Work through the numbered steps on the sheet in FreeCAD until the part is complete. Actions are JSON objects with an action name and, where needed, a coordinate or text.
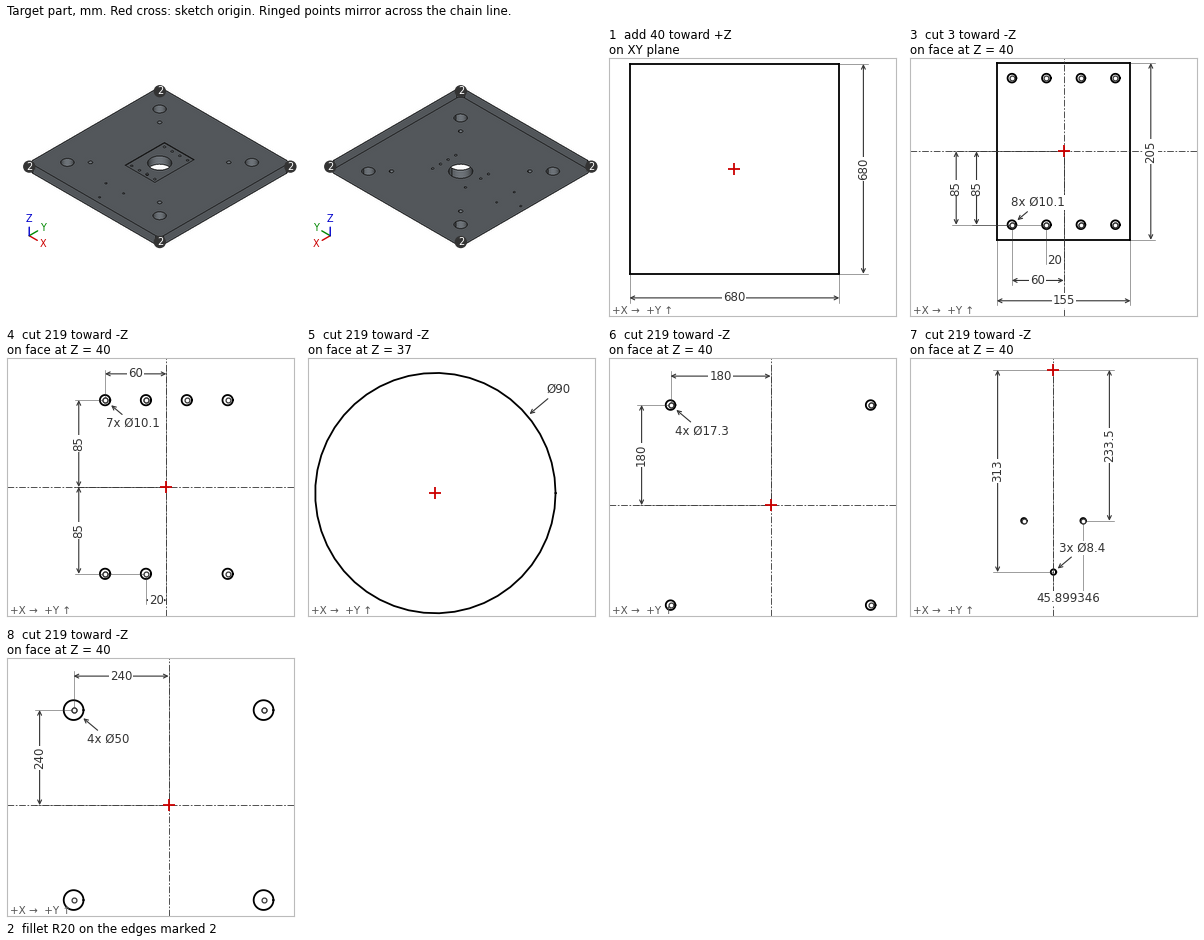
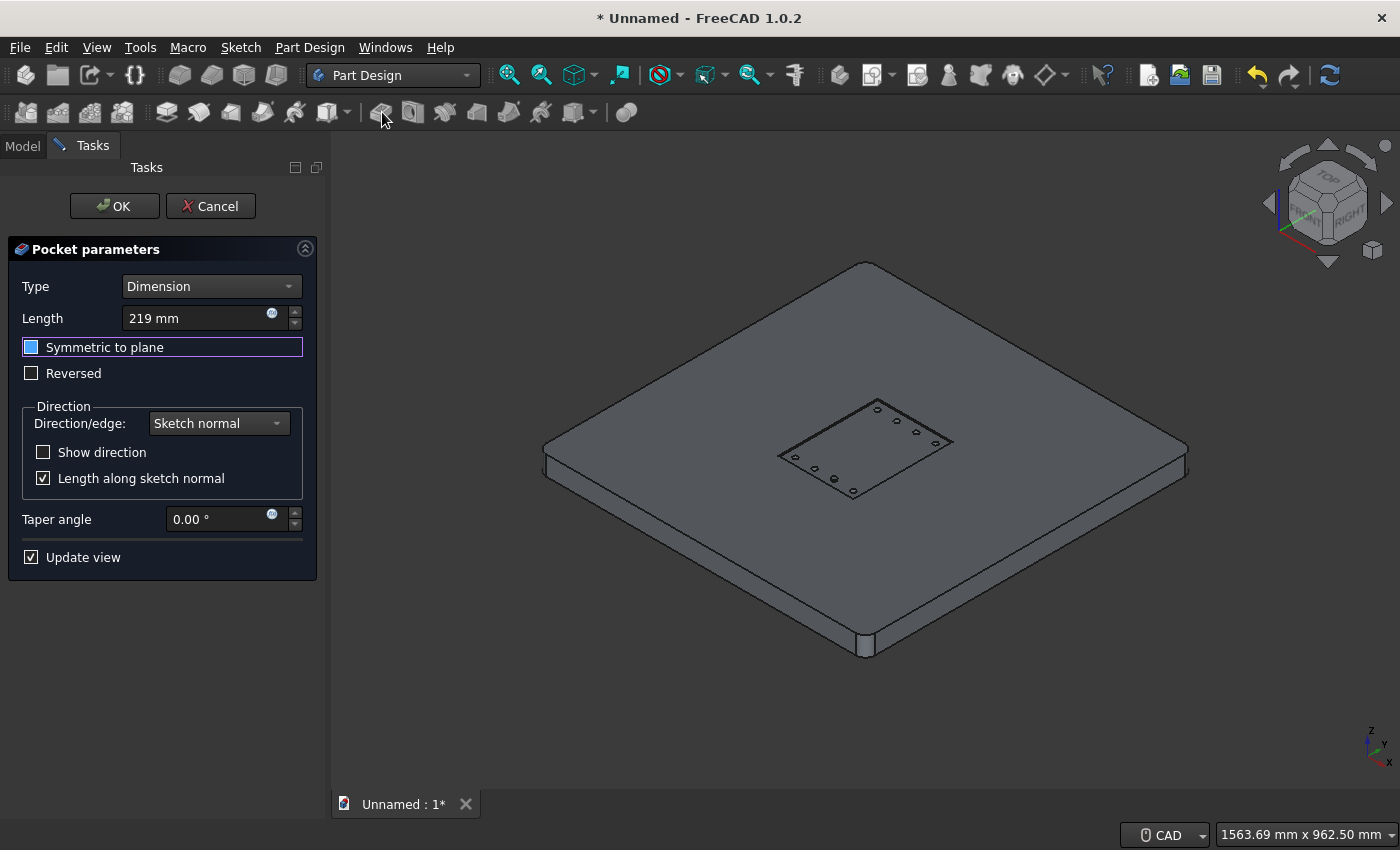
{"action": "left_click", "coordinate": [115, 206]}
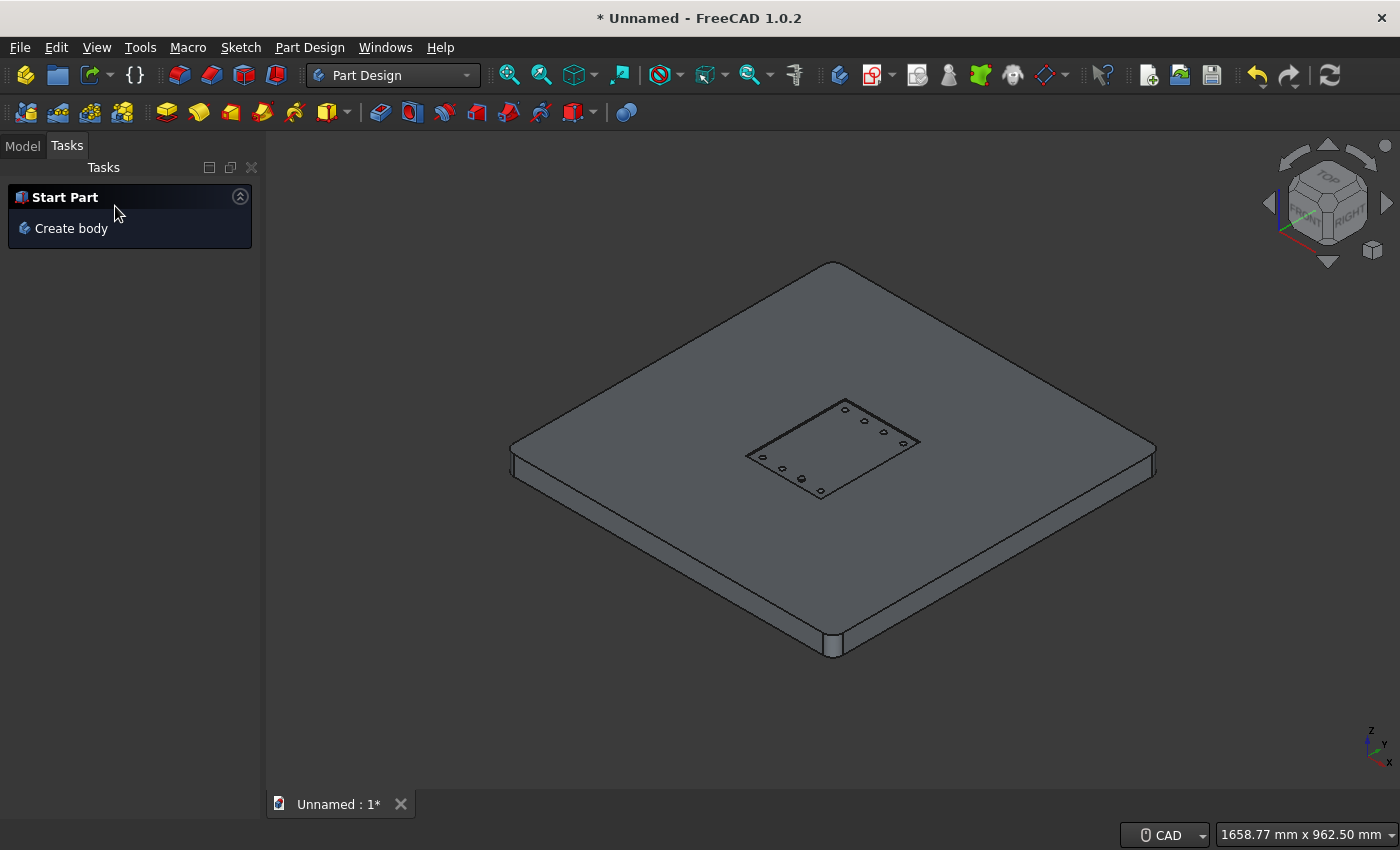
{"action": "left_click", "coordinate": [833, 450]}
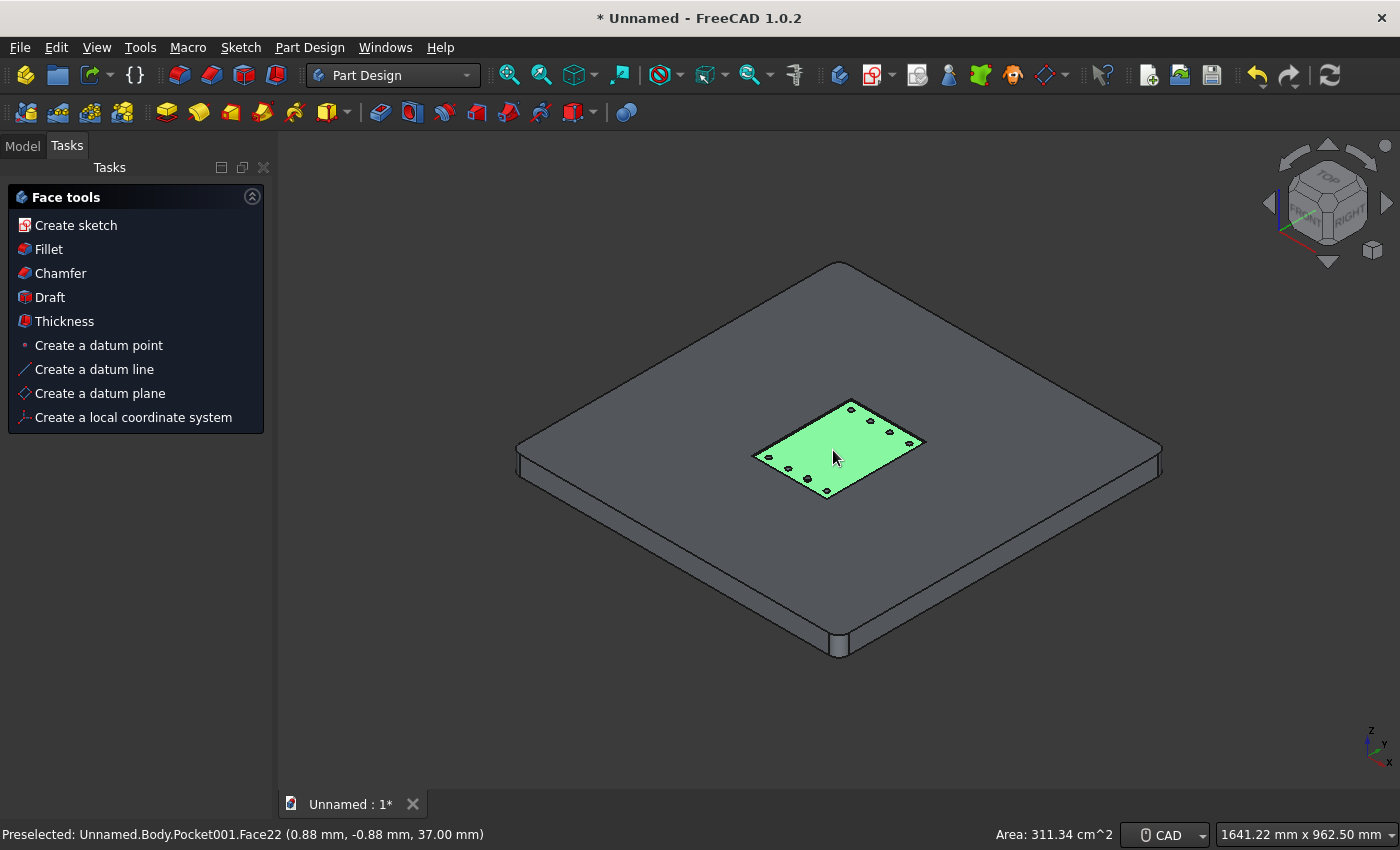
{"action": "left_click", "coordinate": [872, 76]}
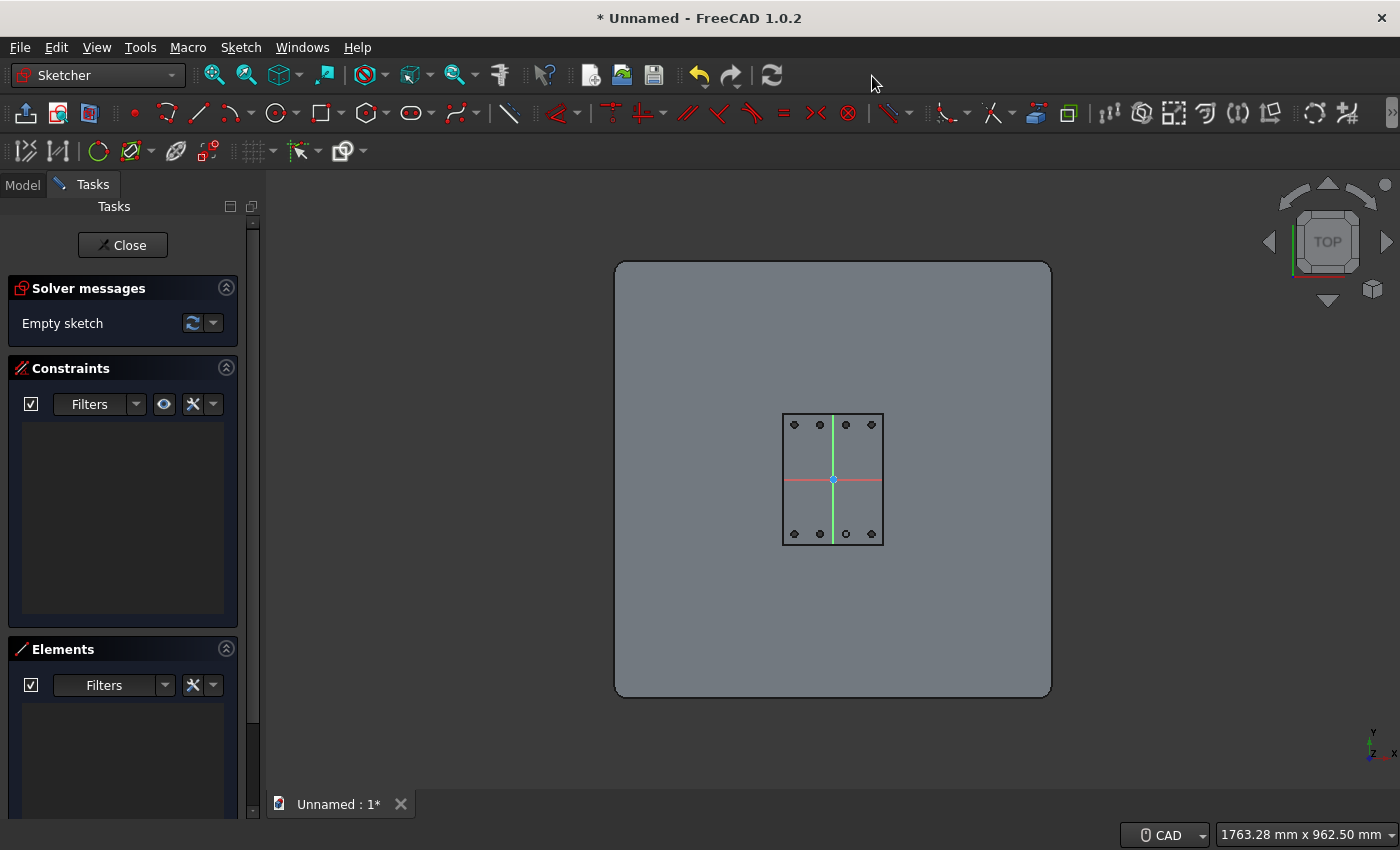
{"action": "left_click", "coordinate": [90, 114]}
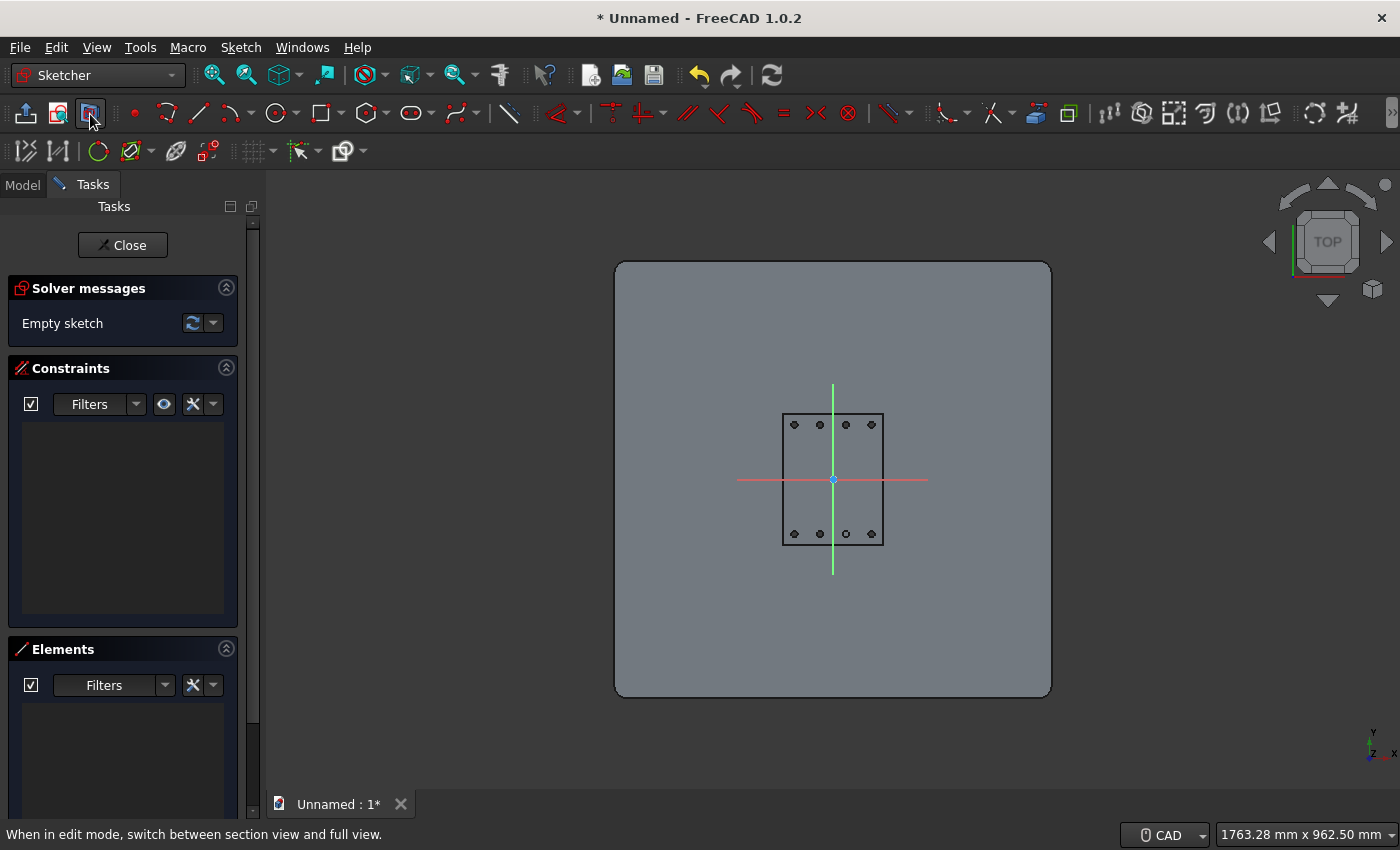
{"action": "scroll", "coordinate": [844, 479], "scroll_direction": "up", "scroll_amount": 10}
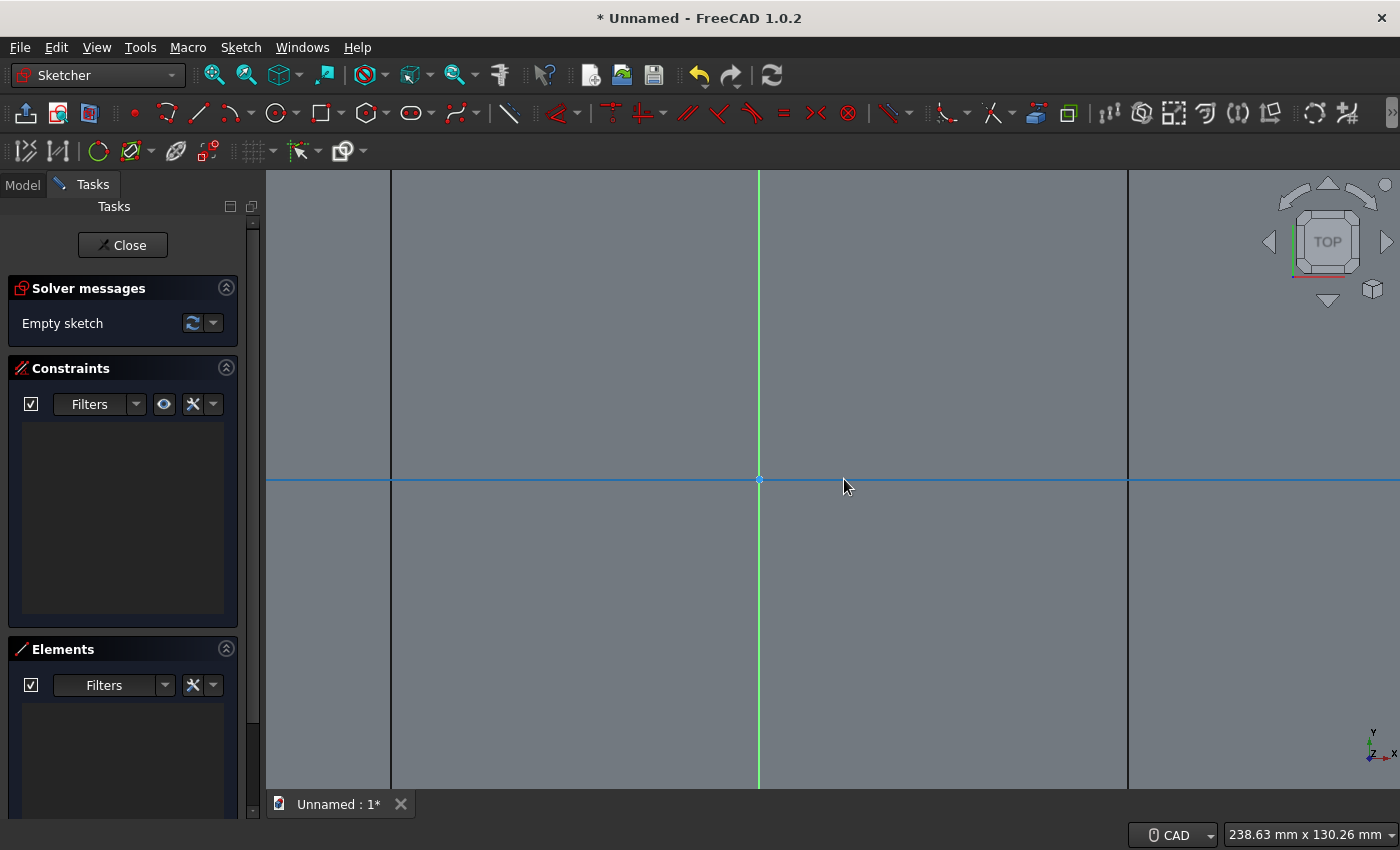
{"action": "left_click", "coordinate": [276, 114]}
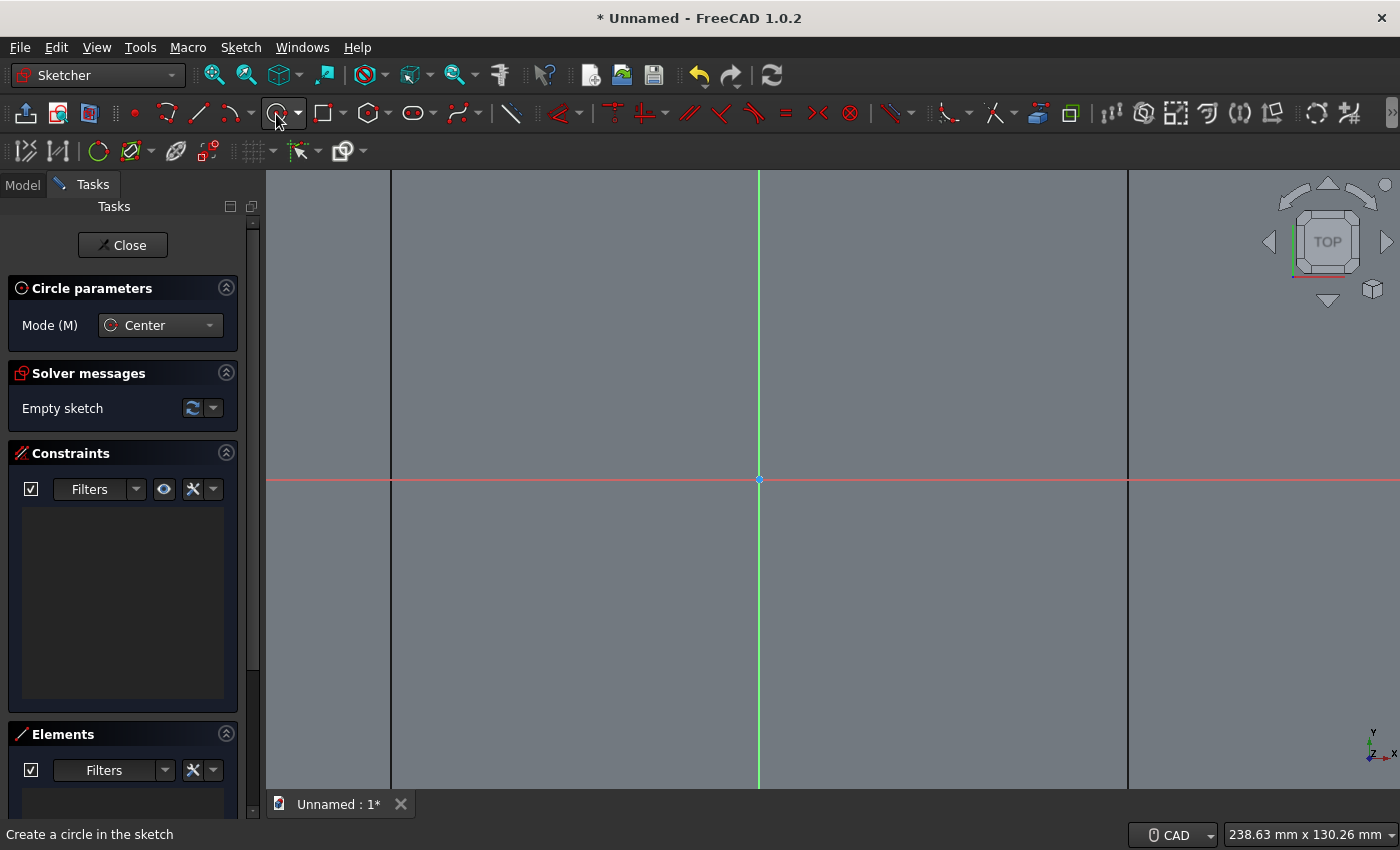
{"action": "left_click", "coordinate": [759, 479]}
{"action": "left_click", "coordinate": [911, 328]}
{"action": "key", "text": "Escape"}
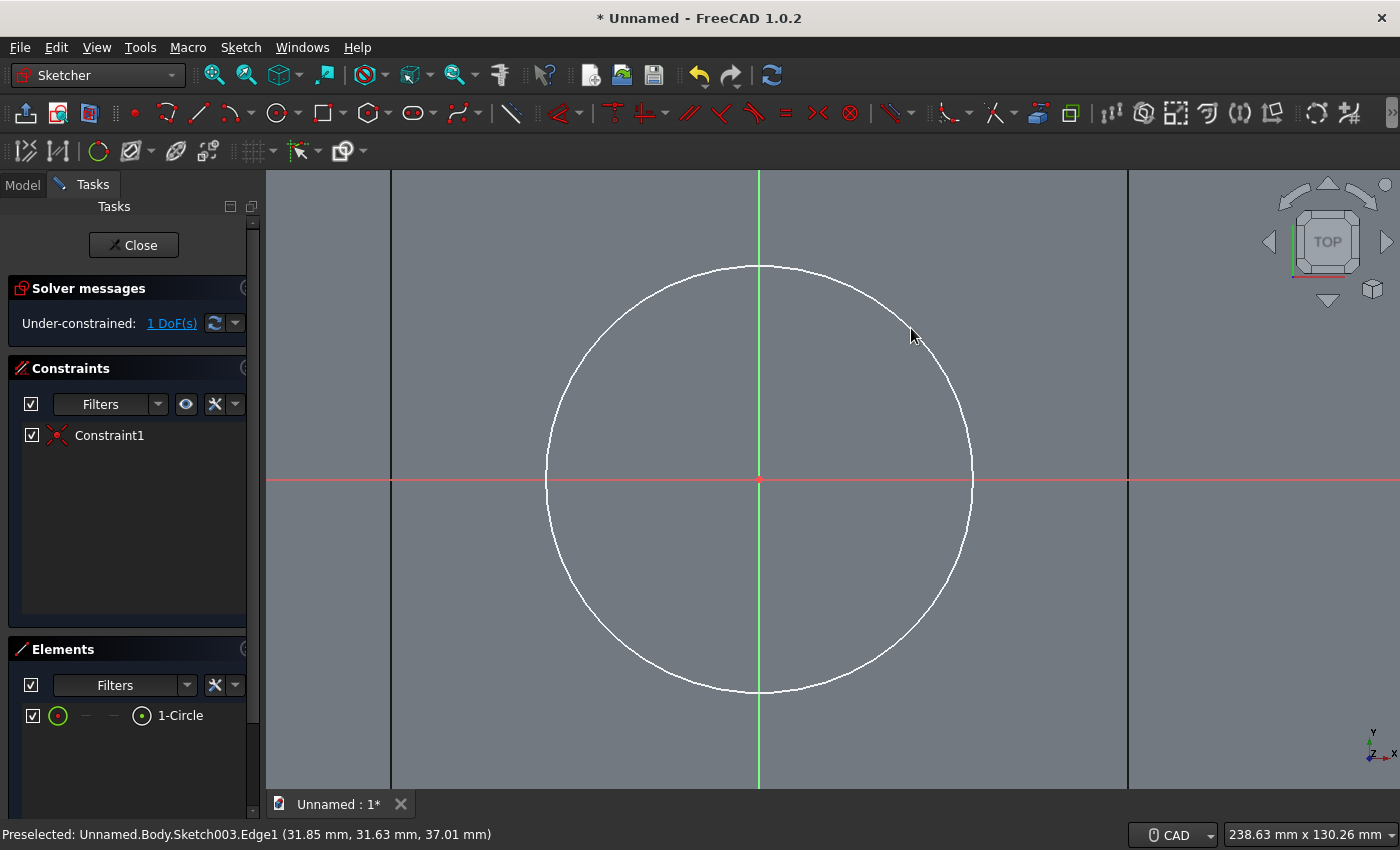
{"action": "left_click", "coordinate": [558, 114]}